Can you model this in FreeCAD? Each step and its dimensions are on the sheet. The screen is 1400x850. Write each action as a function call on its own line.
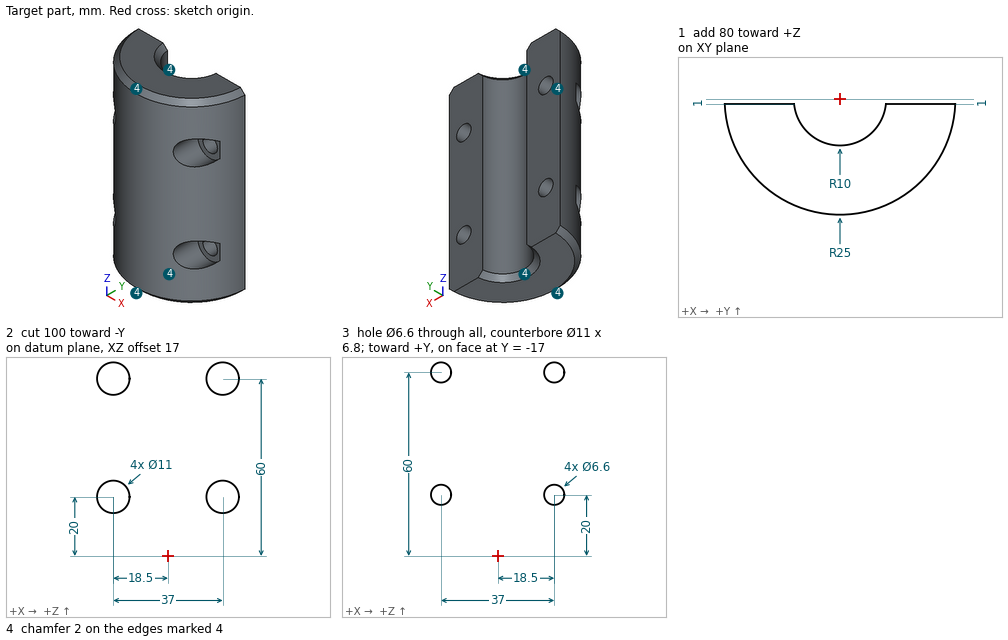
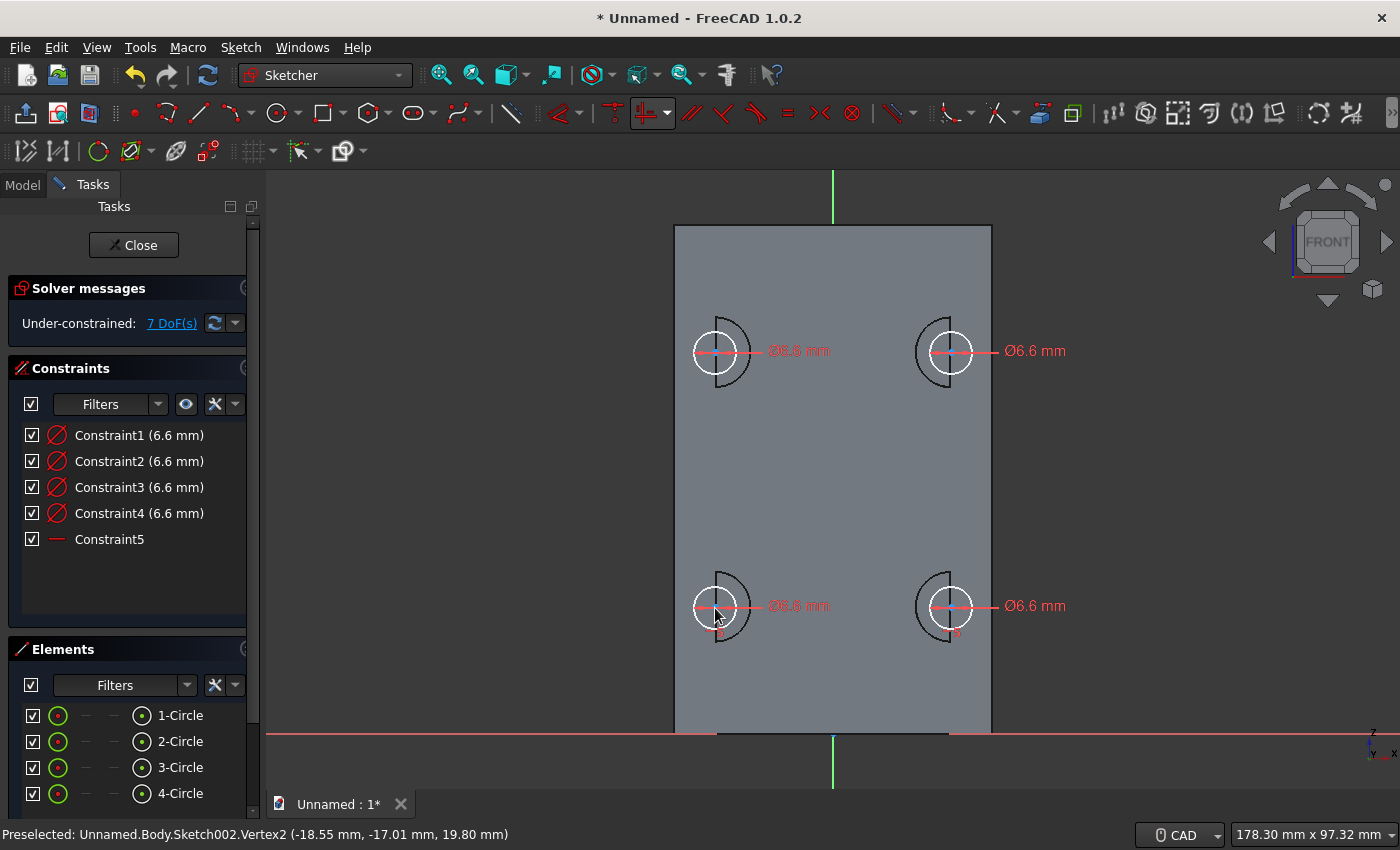
click(715, 608)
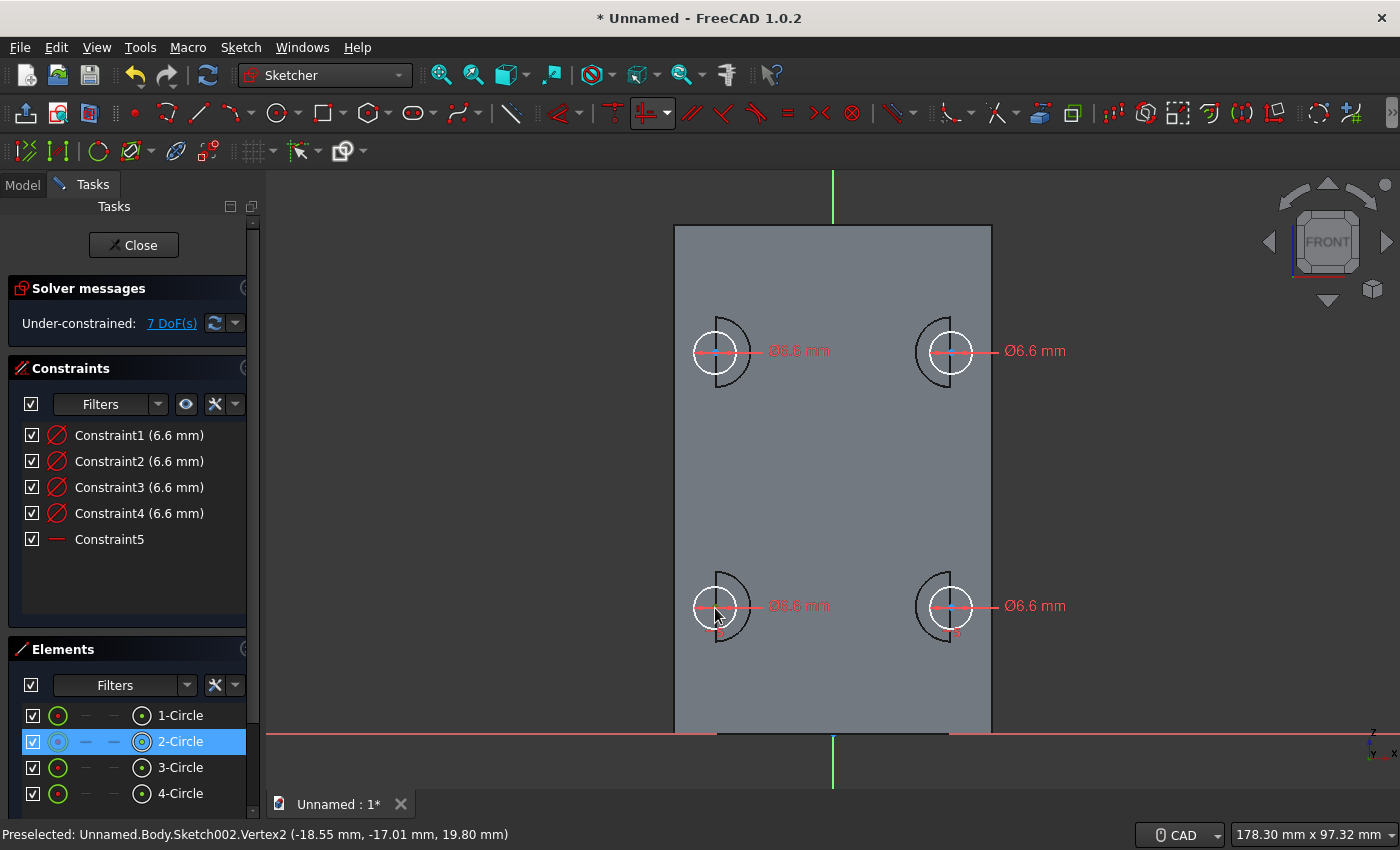
click(715, 353)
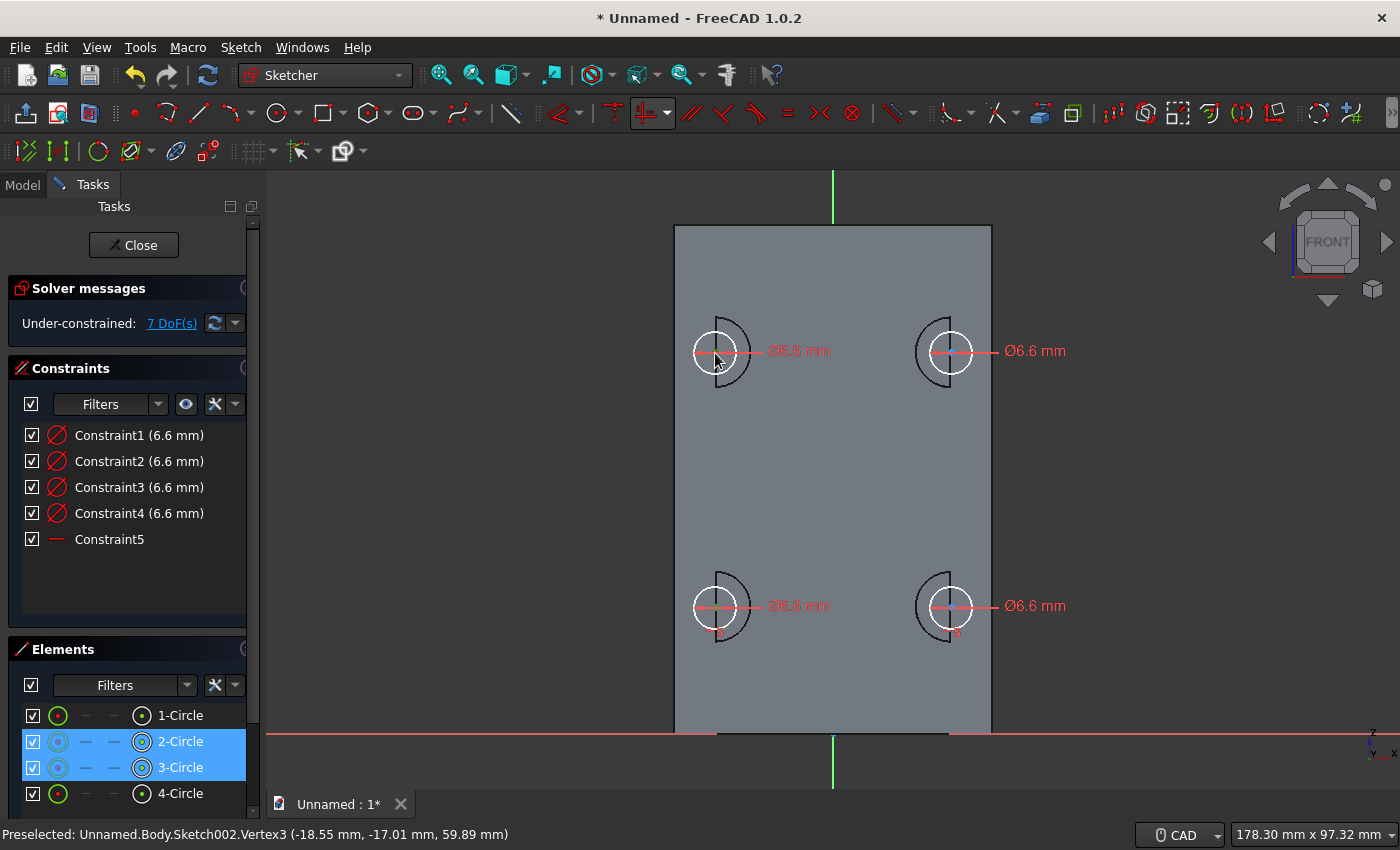
key(v)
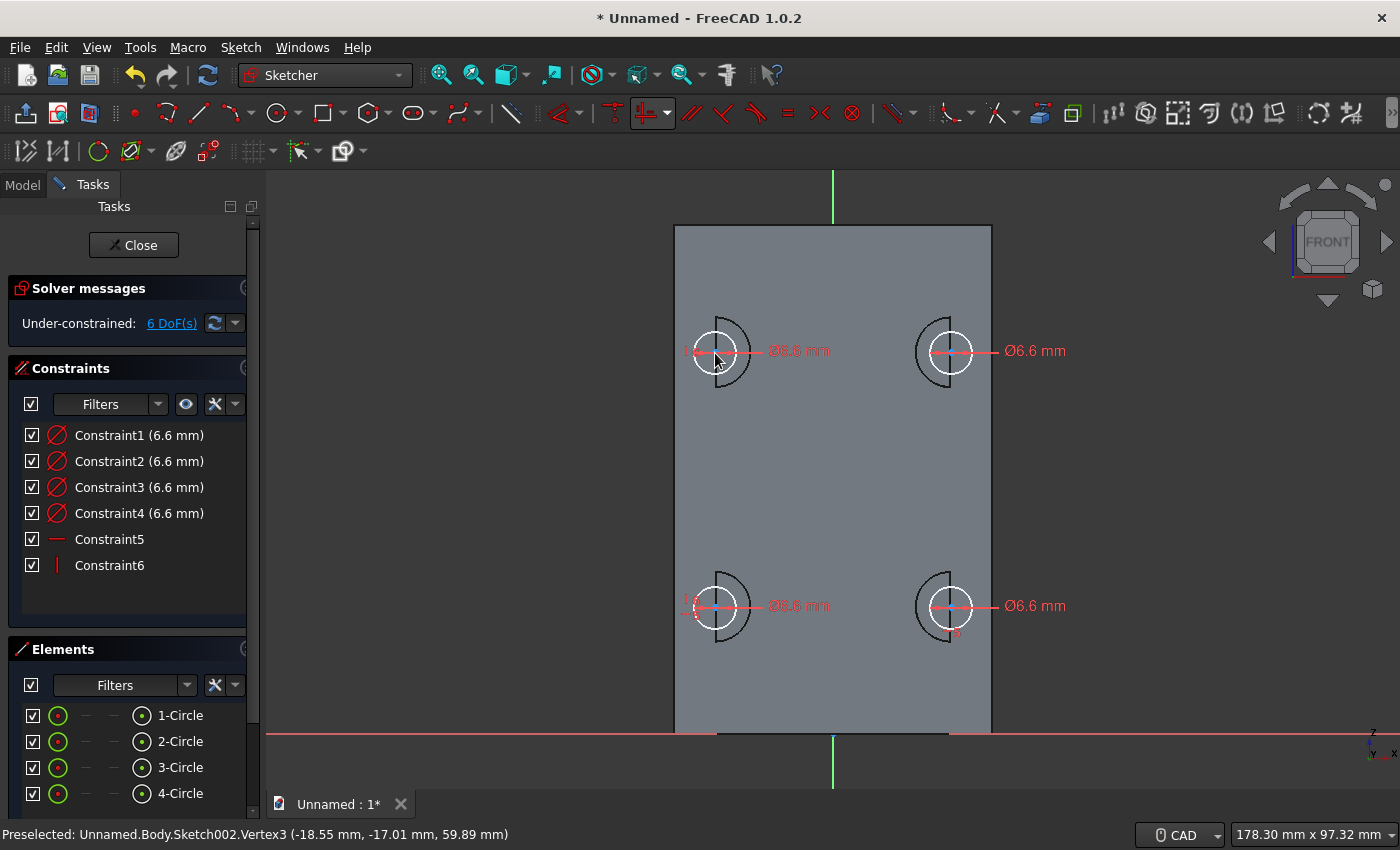
click(951, 608)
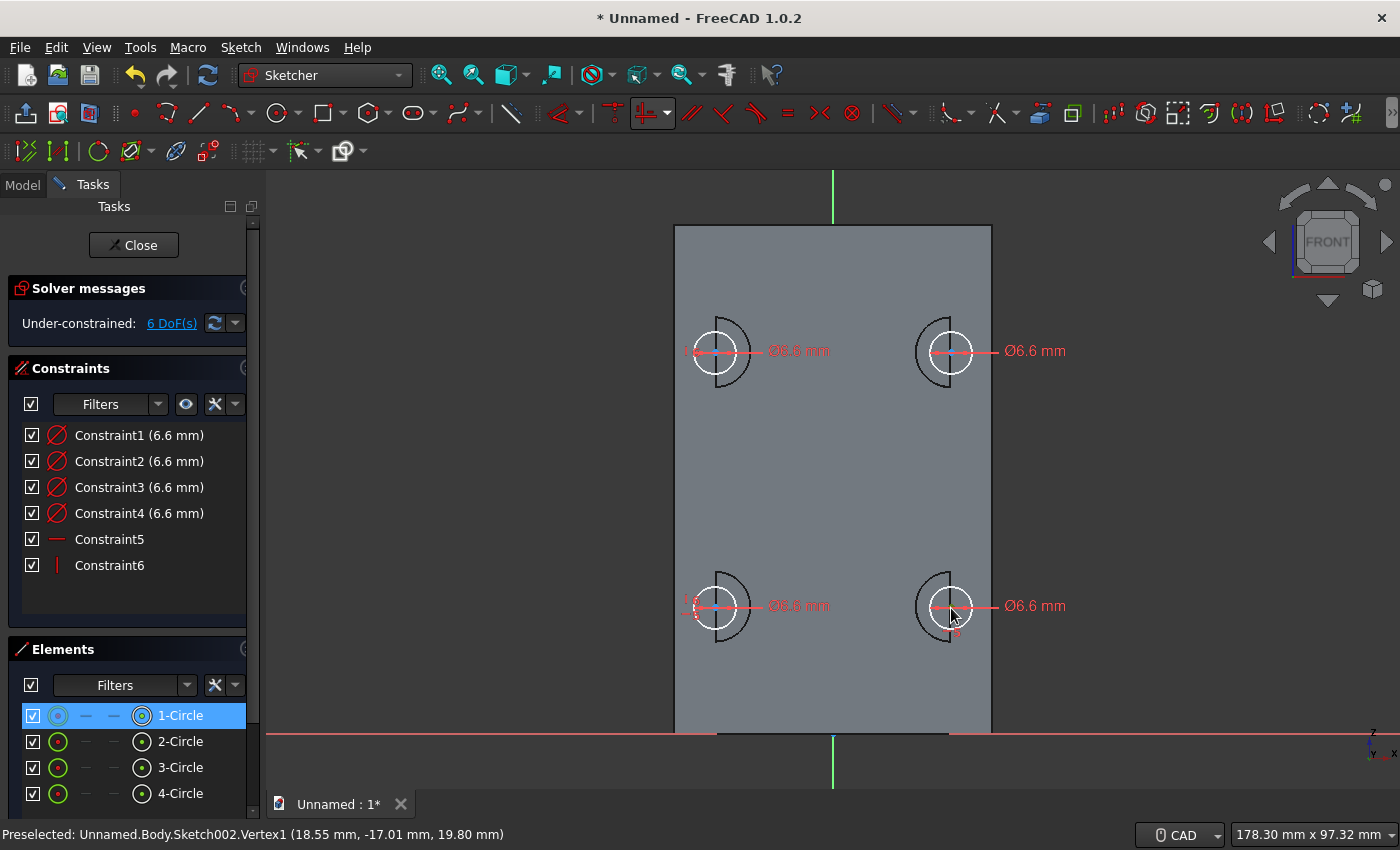
click(951, 353)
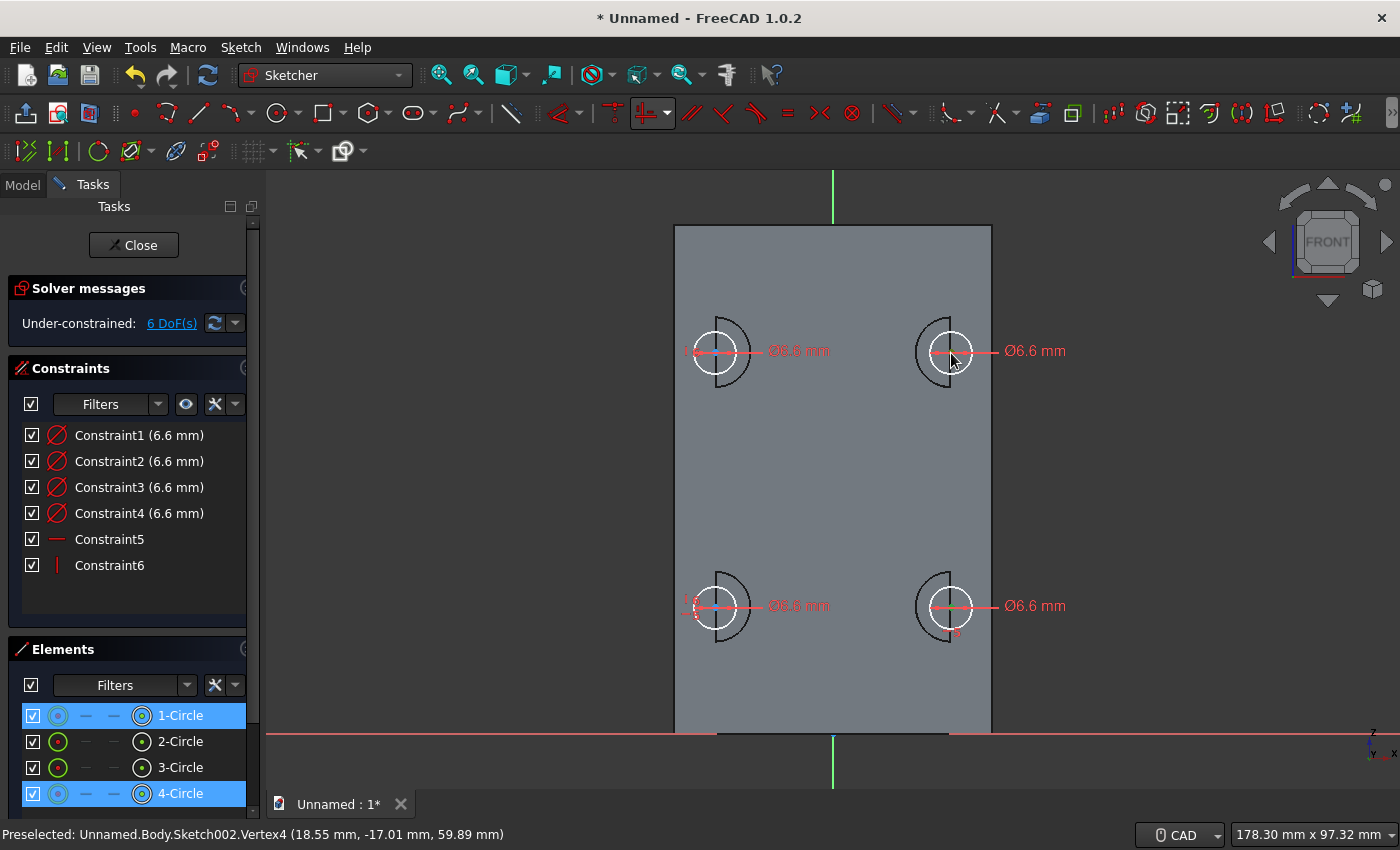
click(670, 114)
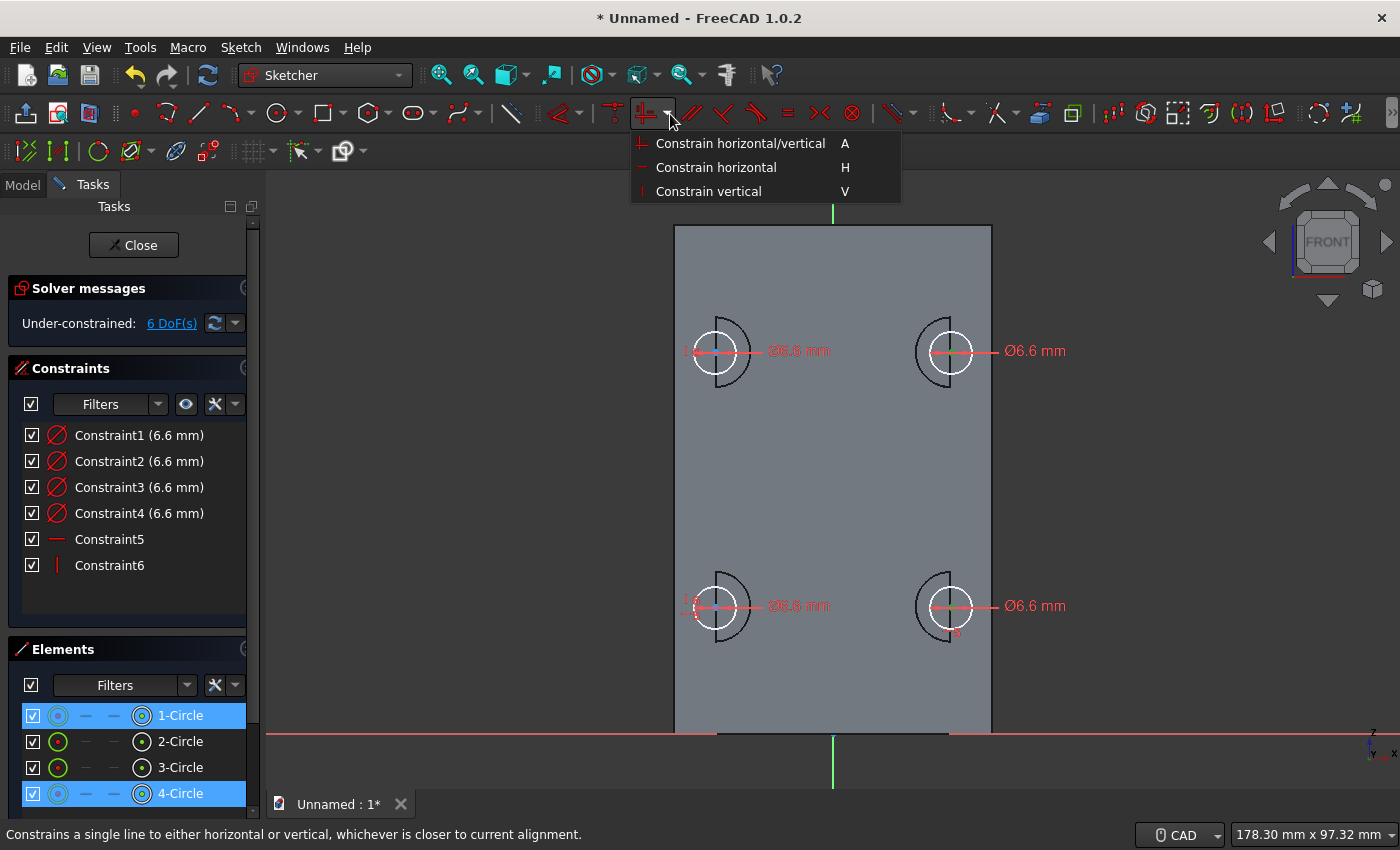
click(766, 191)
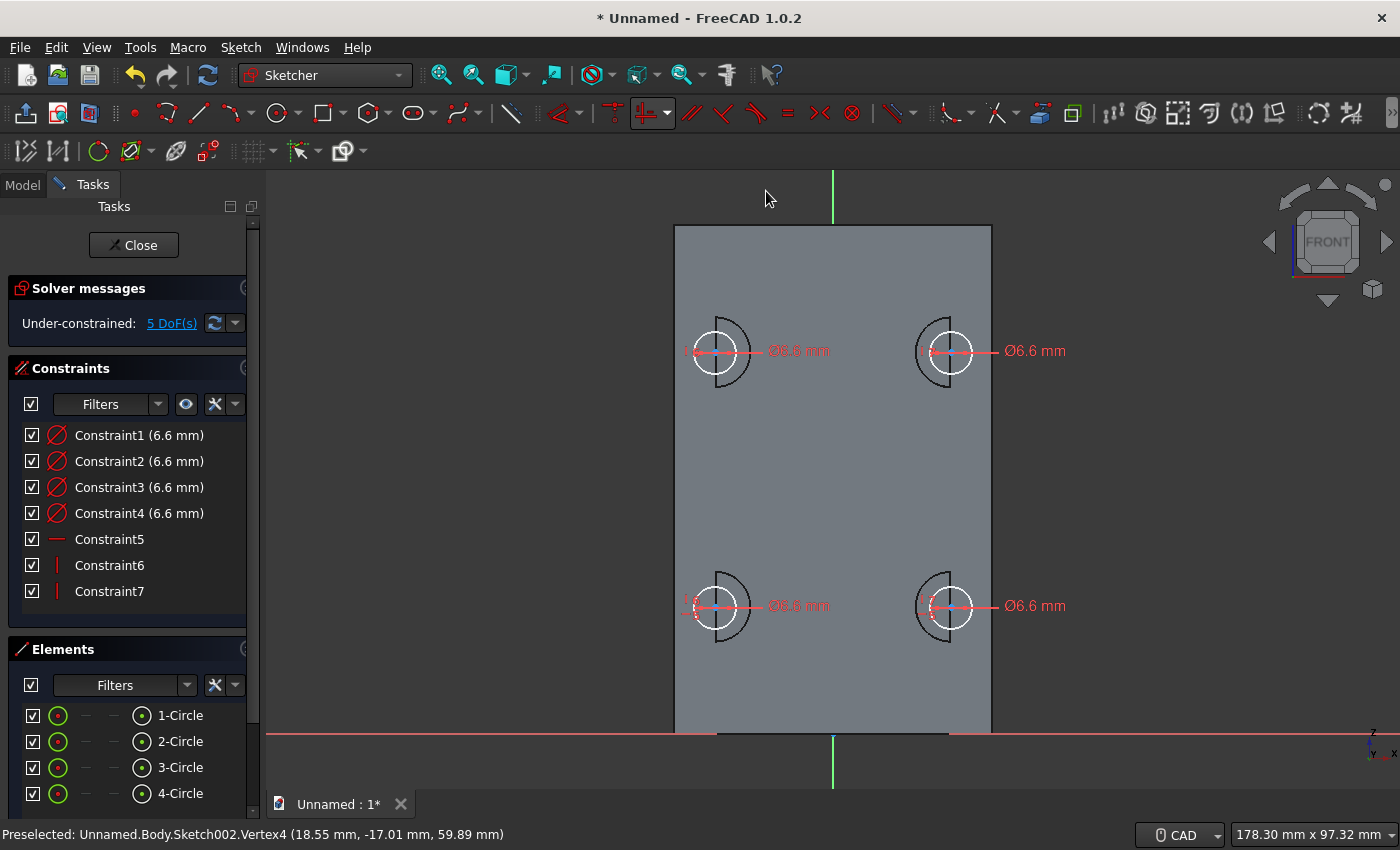
click(715, 353)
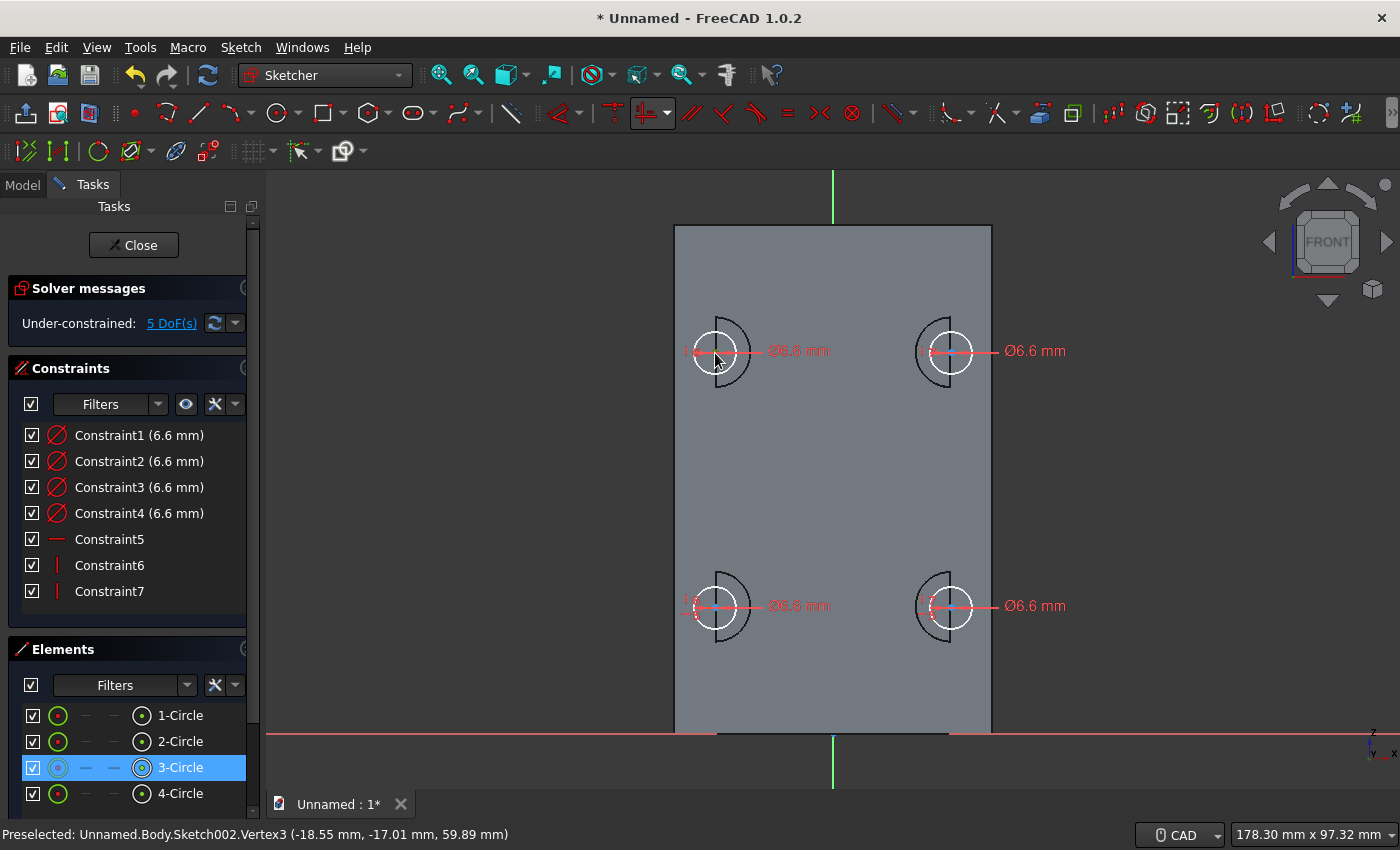
click(951, 353)